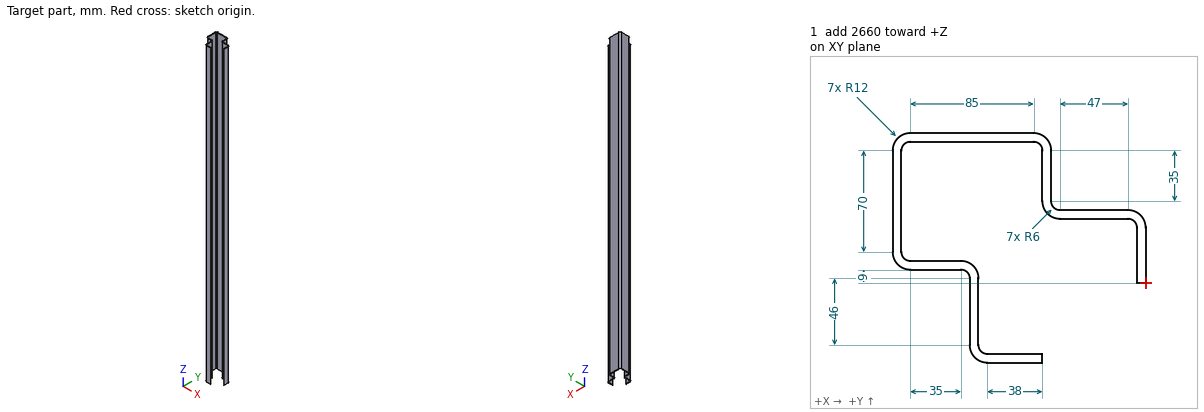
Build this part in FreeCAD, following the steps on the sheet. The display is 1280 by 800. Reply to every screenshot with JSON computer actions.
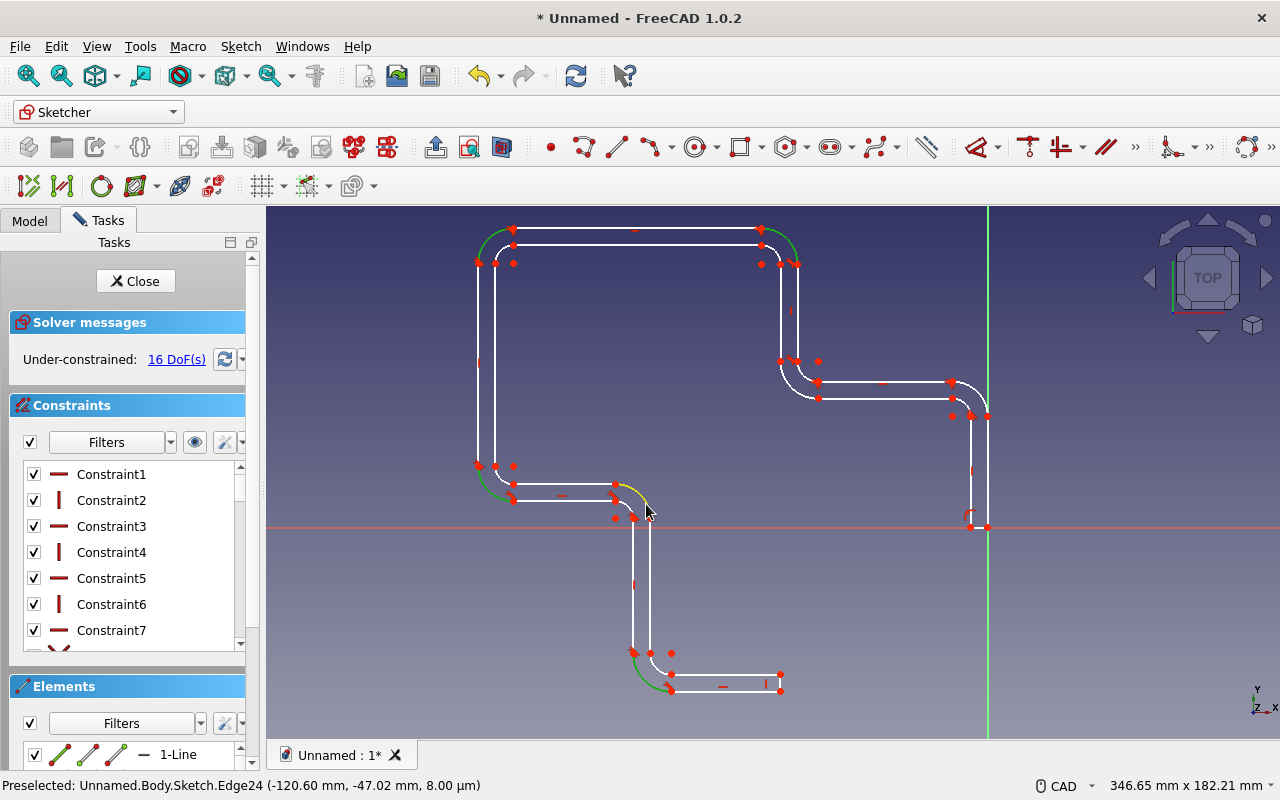
{"action": "left_click", "coordinate": [646, 503]}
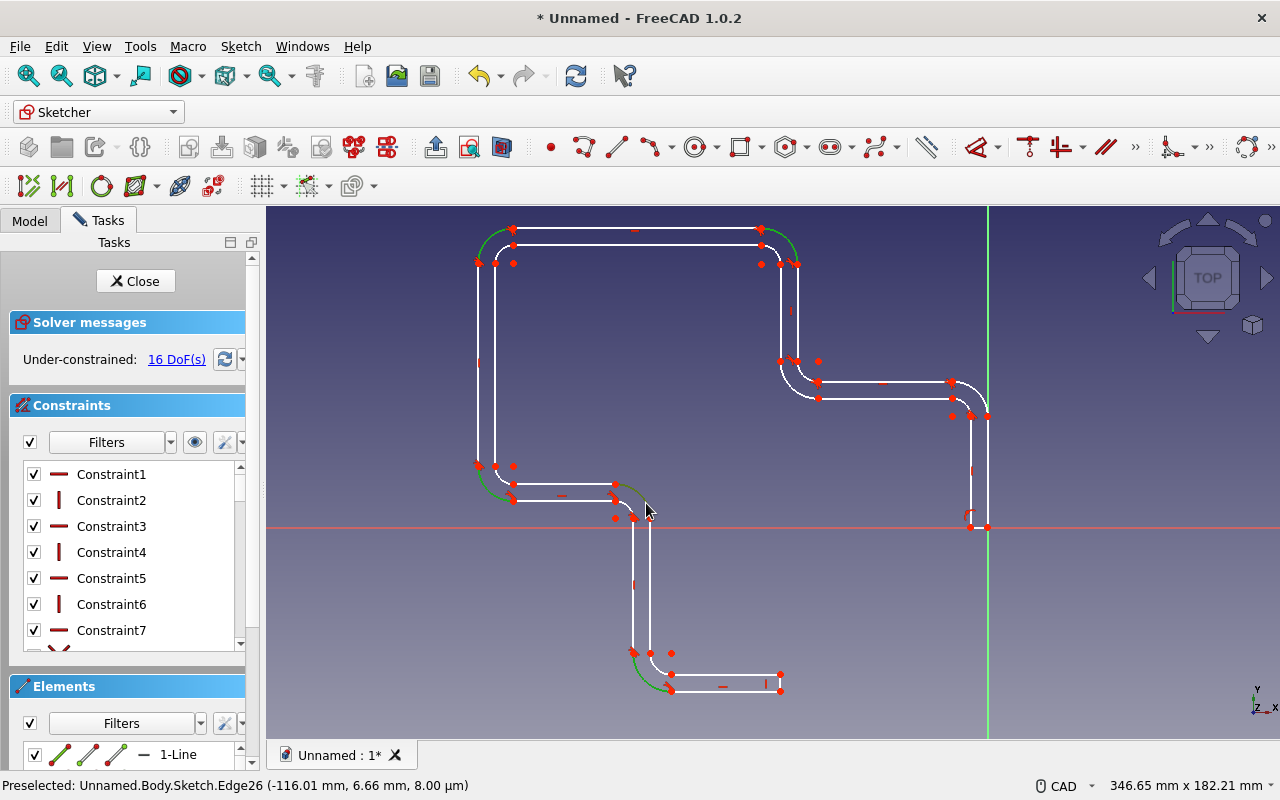
{"action": "left_click", "coordinate": [785, 378]}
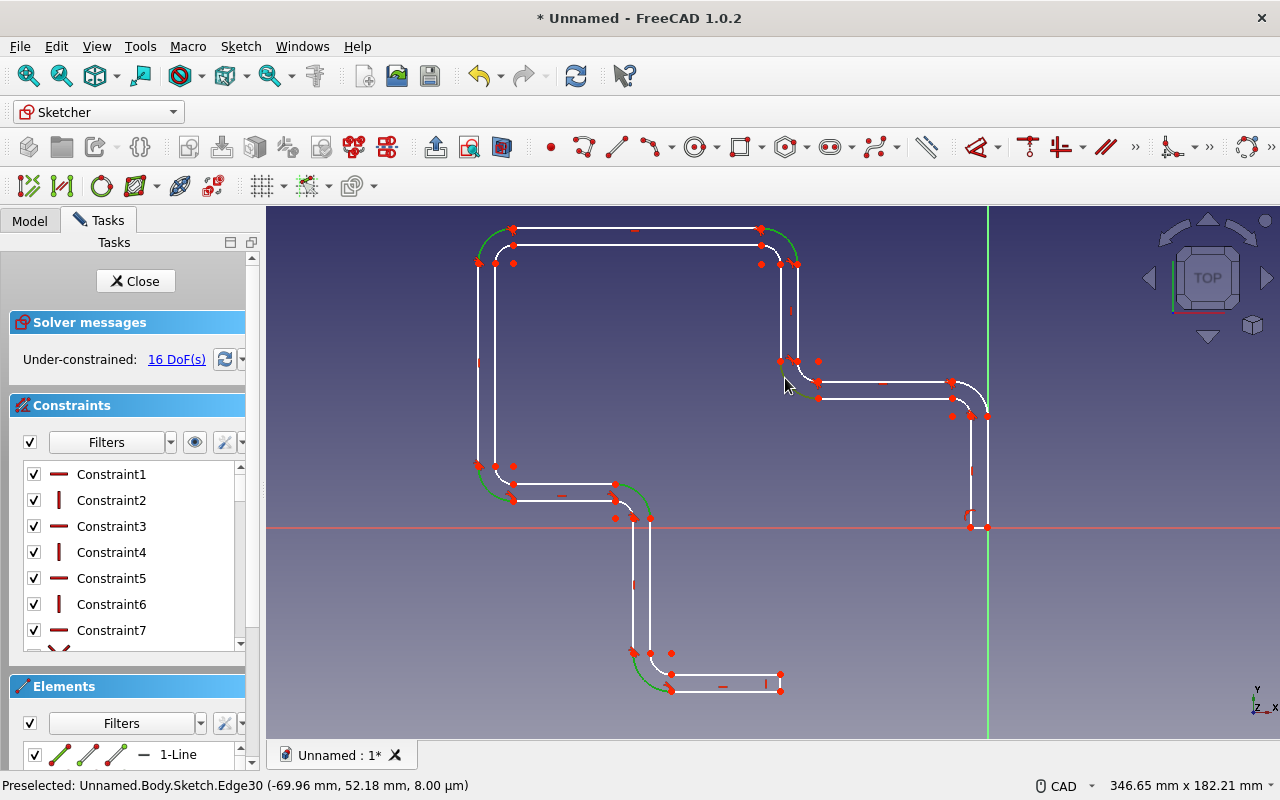
{"action": "left_click", "coordinate": [984, 401]}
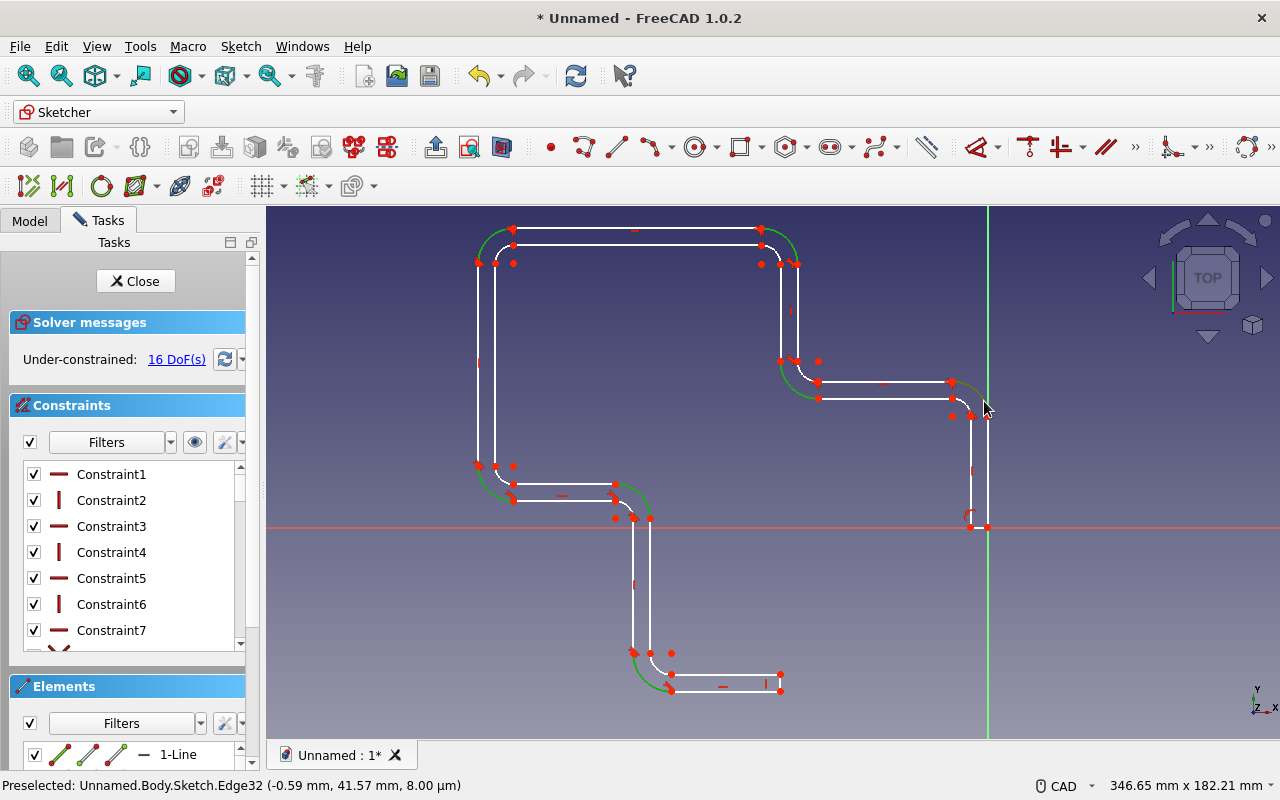
{"action": "key", "text": "e"}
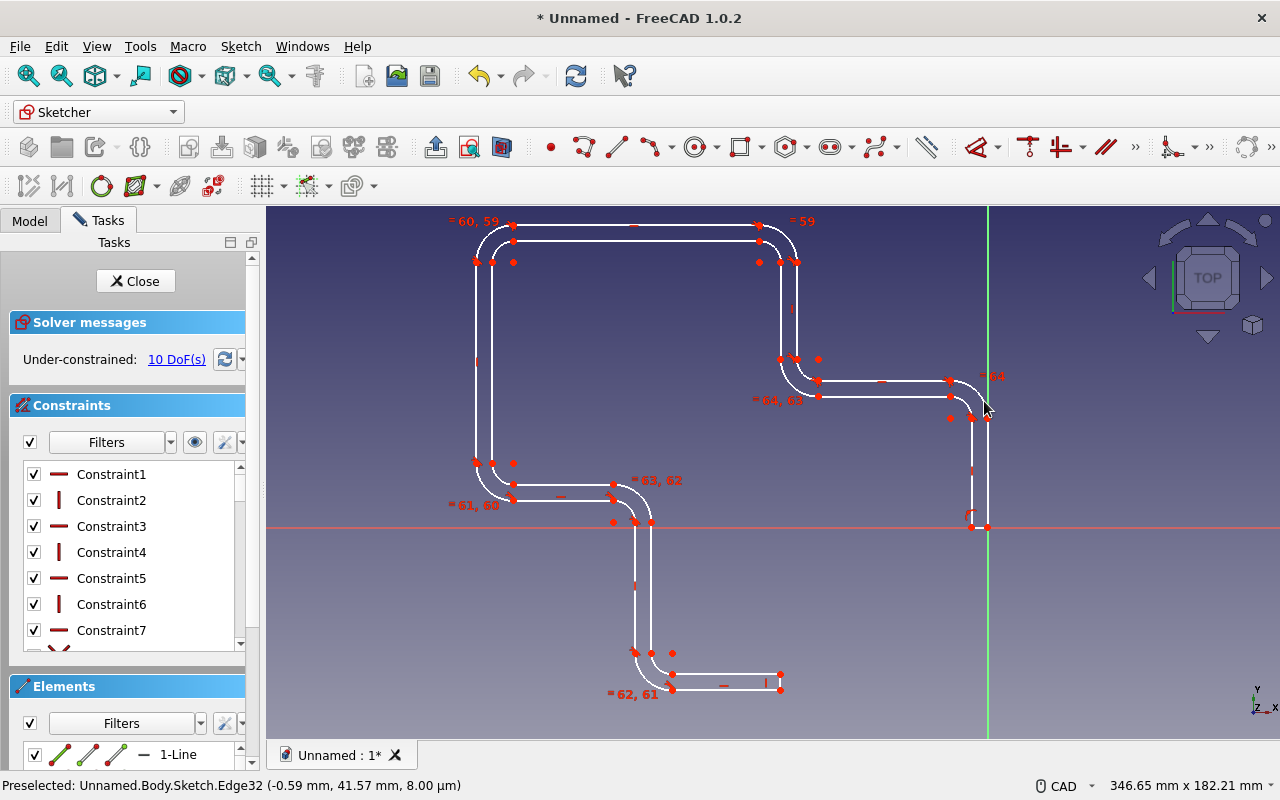
{"action": "key", "text": "d"}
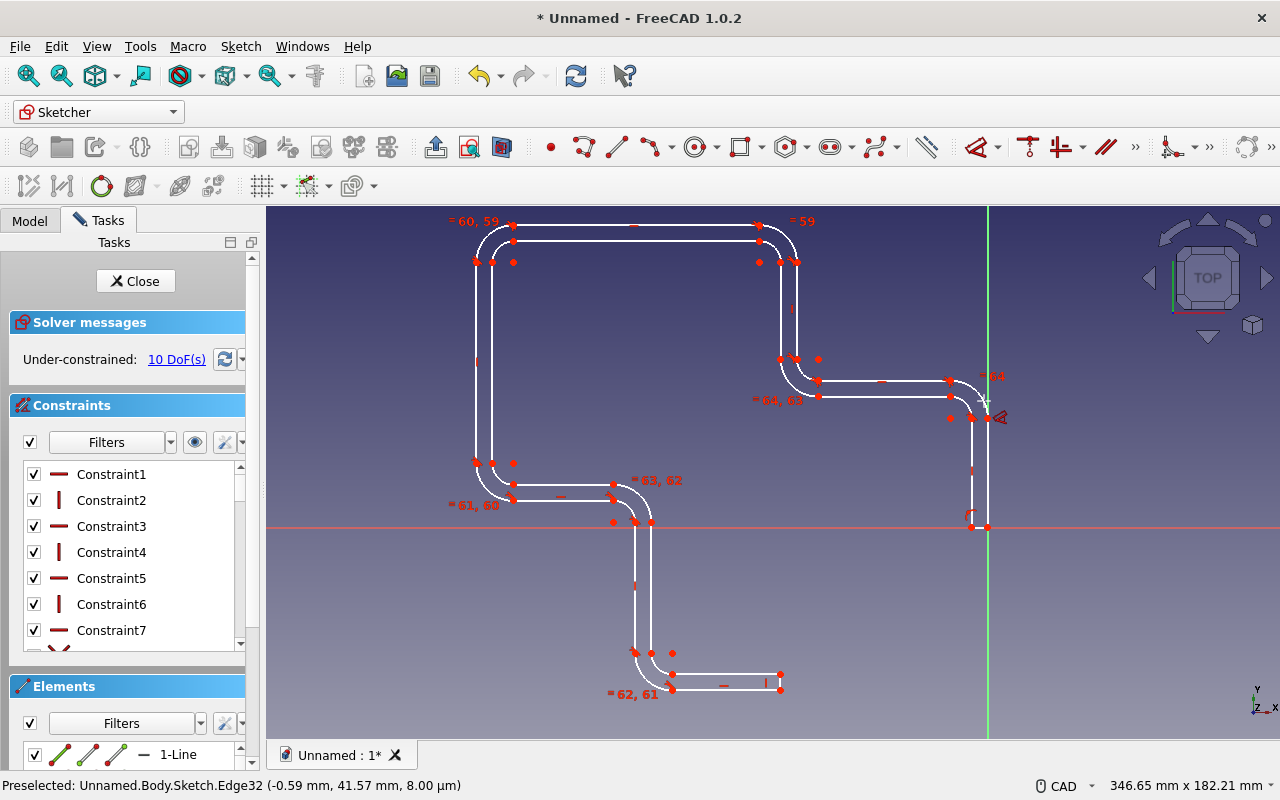
{"action": "scroll", "coordinate": [799, 369], "scroll_direction": "up", "scroll_amount": 5}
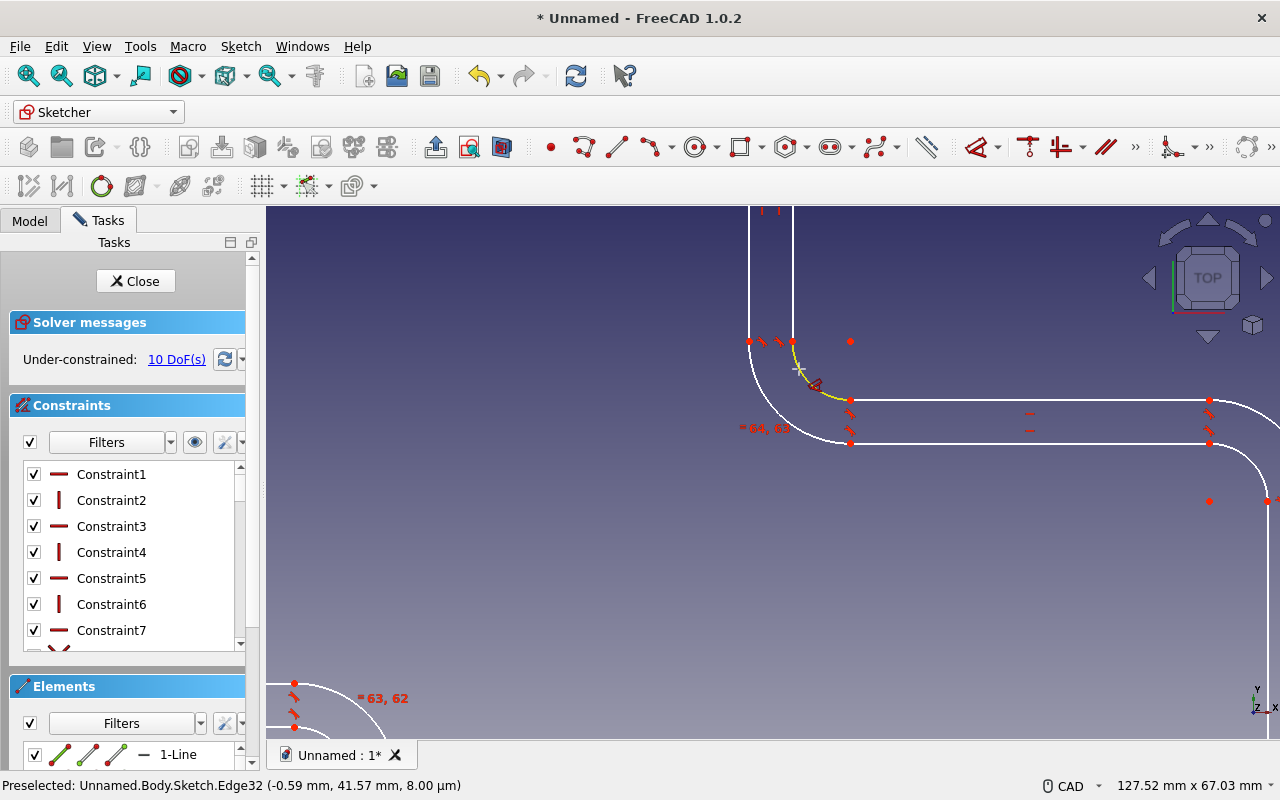
{"action": "left_click", "coordinate": [799, 368]}
{"action": "left_click", "coordinate": [773, 296]}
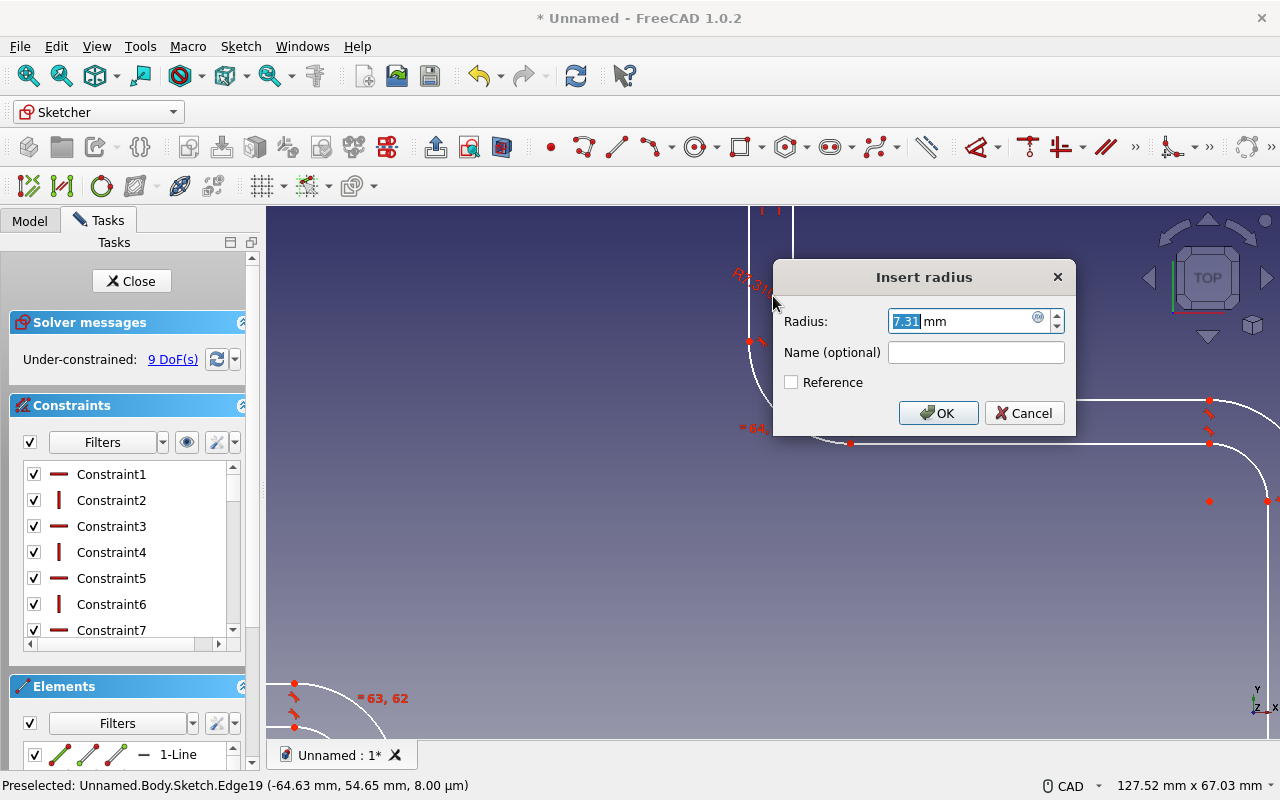
{"action": "type", "text": "6"}
{"action": "key", "text": "Return"}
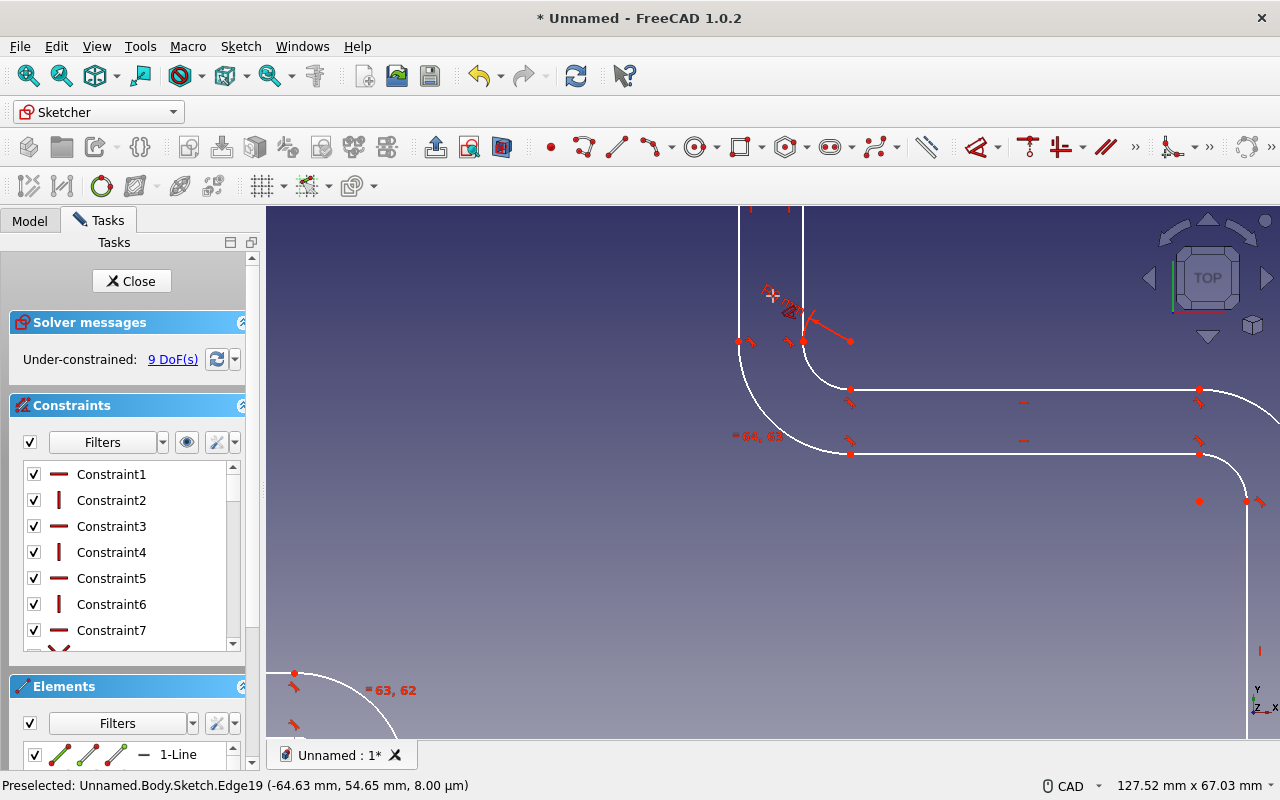
{"action": "scroll", "coordinate": [732, 428], "scroll_direction": "down", "scroll_amount": 7}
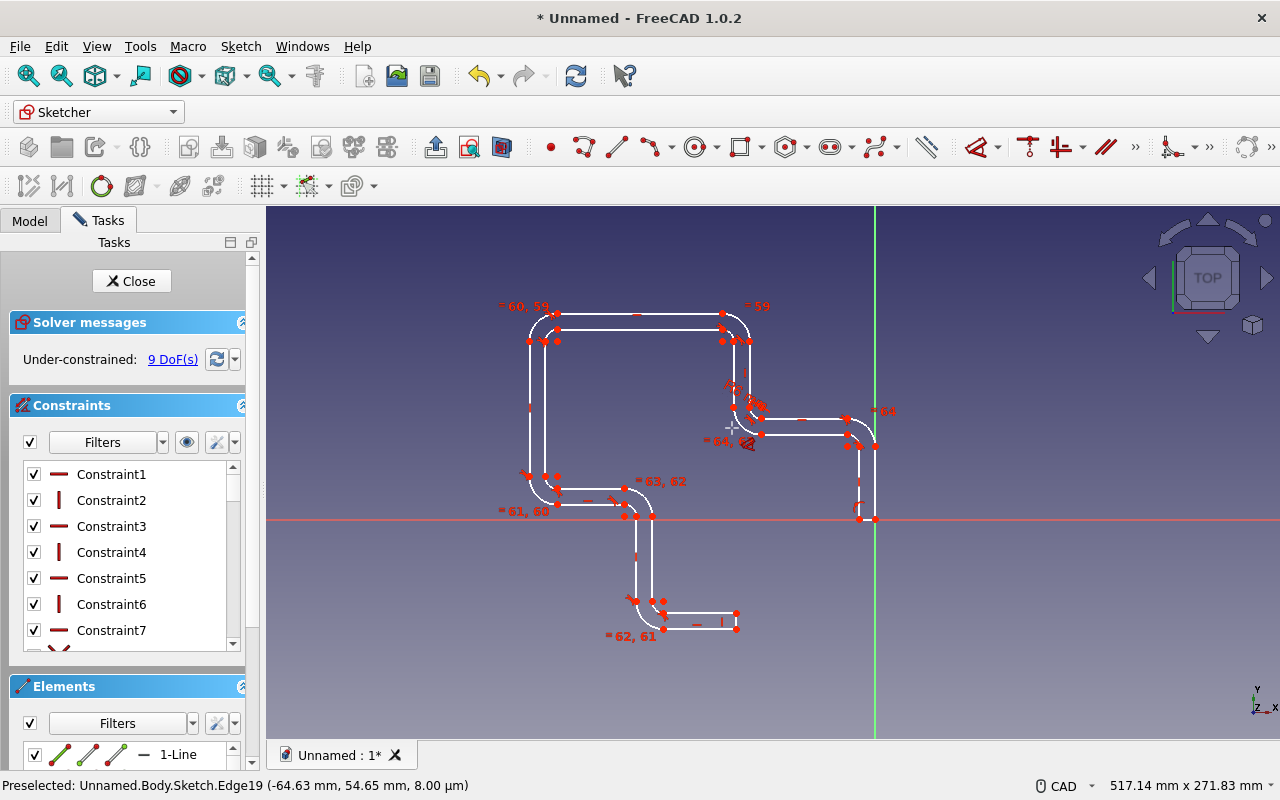
{"action": "scroll", "coordinate": [747, 329], "scroll_direction": "up", "scroll_amount": 3}